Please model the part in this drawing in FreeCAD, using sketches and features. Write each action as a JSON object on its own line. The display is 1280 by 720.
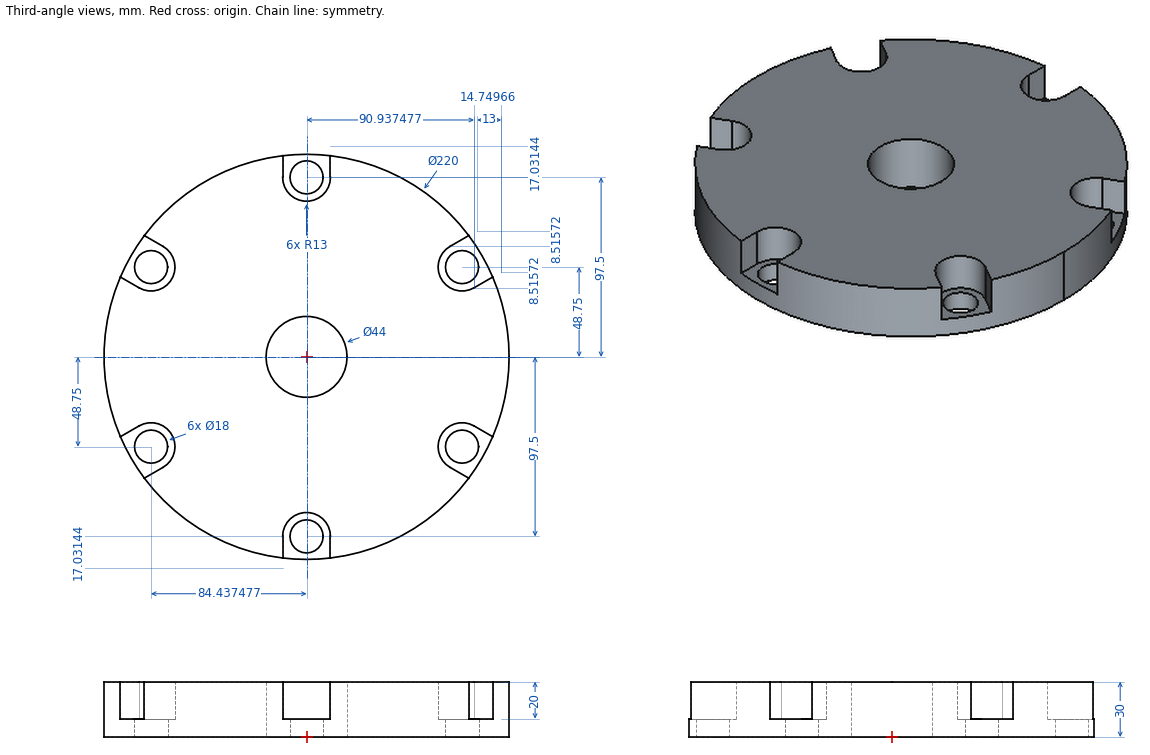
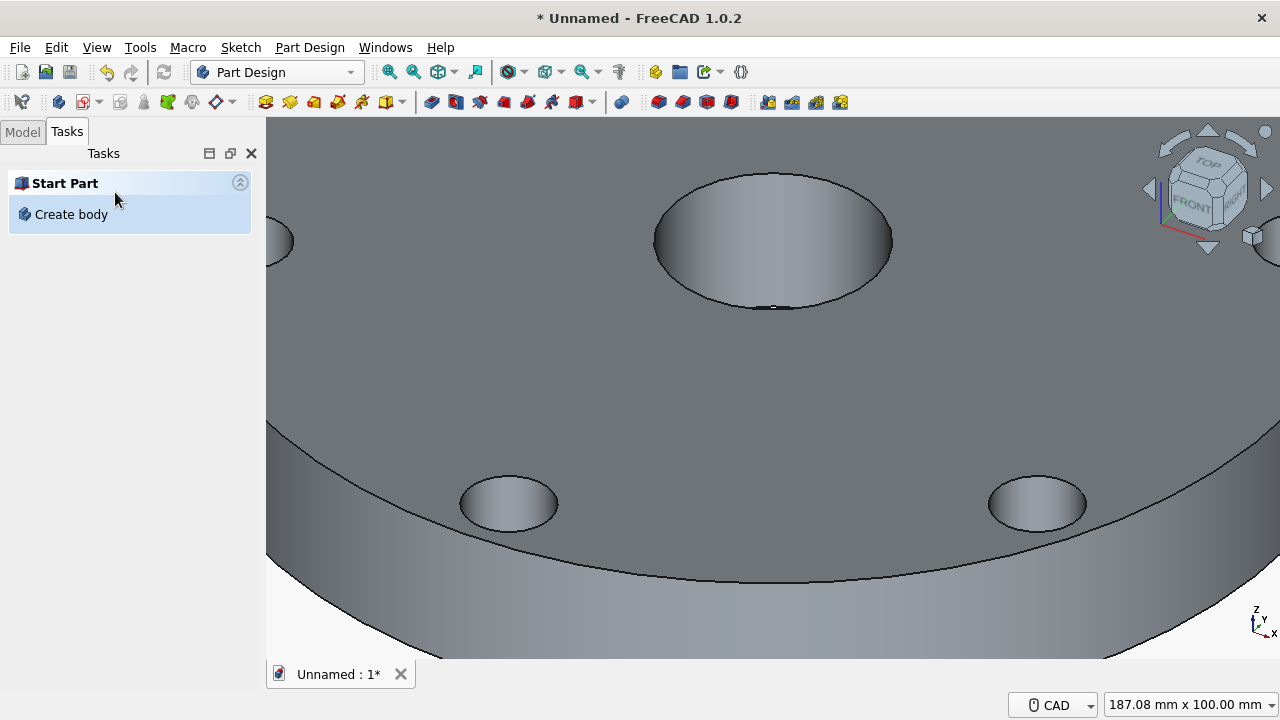
{"action": "key", "text": "v f"}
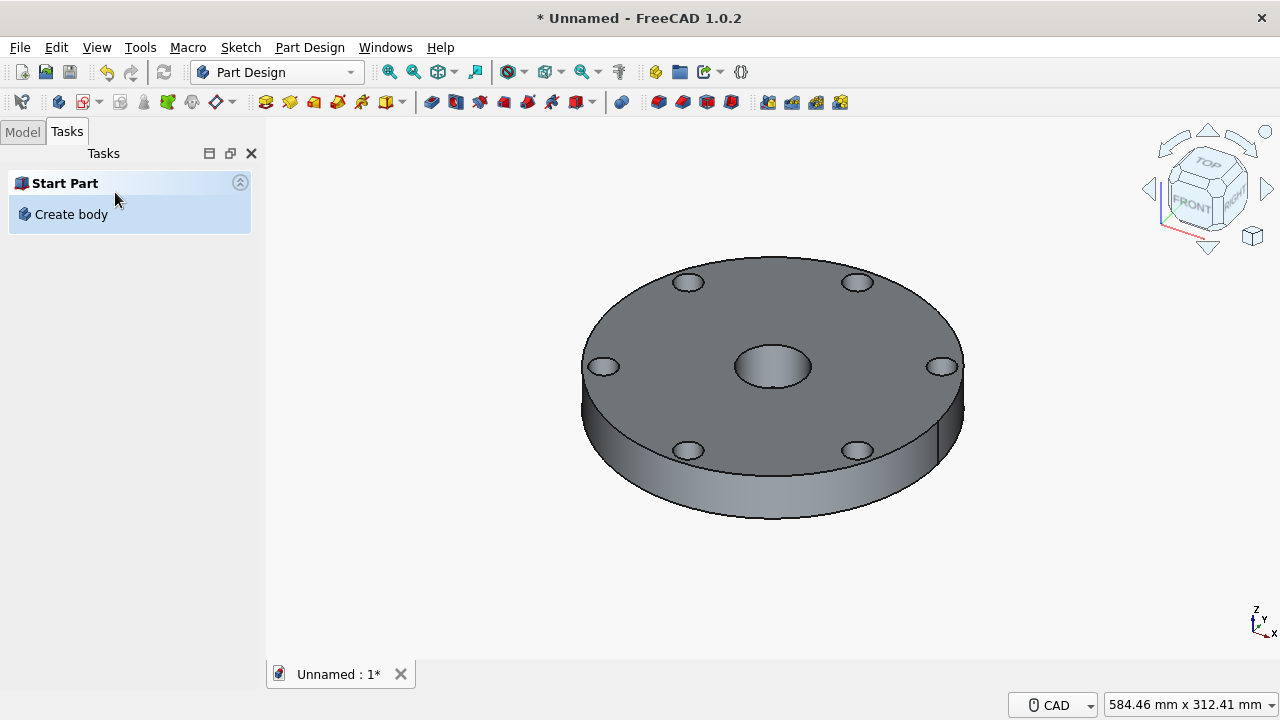
{"action": "left_click", "coordinate": [678, 334]}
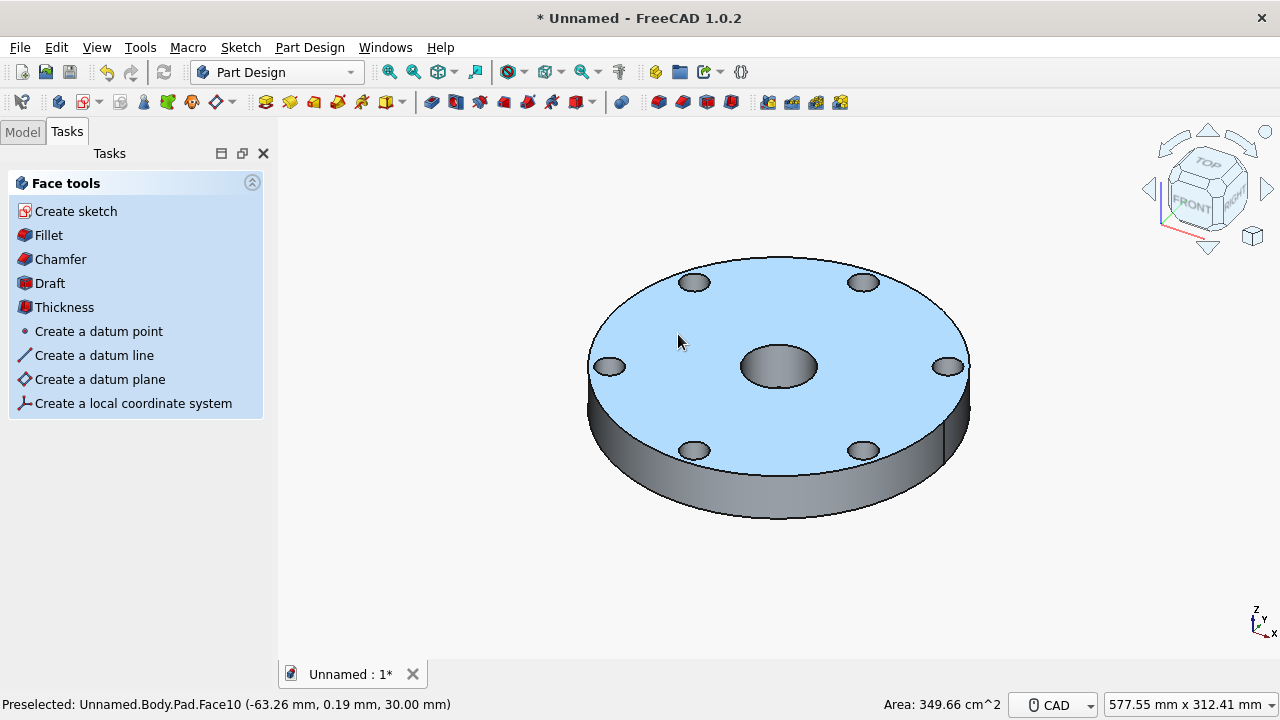
{"action": "left_click", "coordinate": [84, 102]}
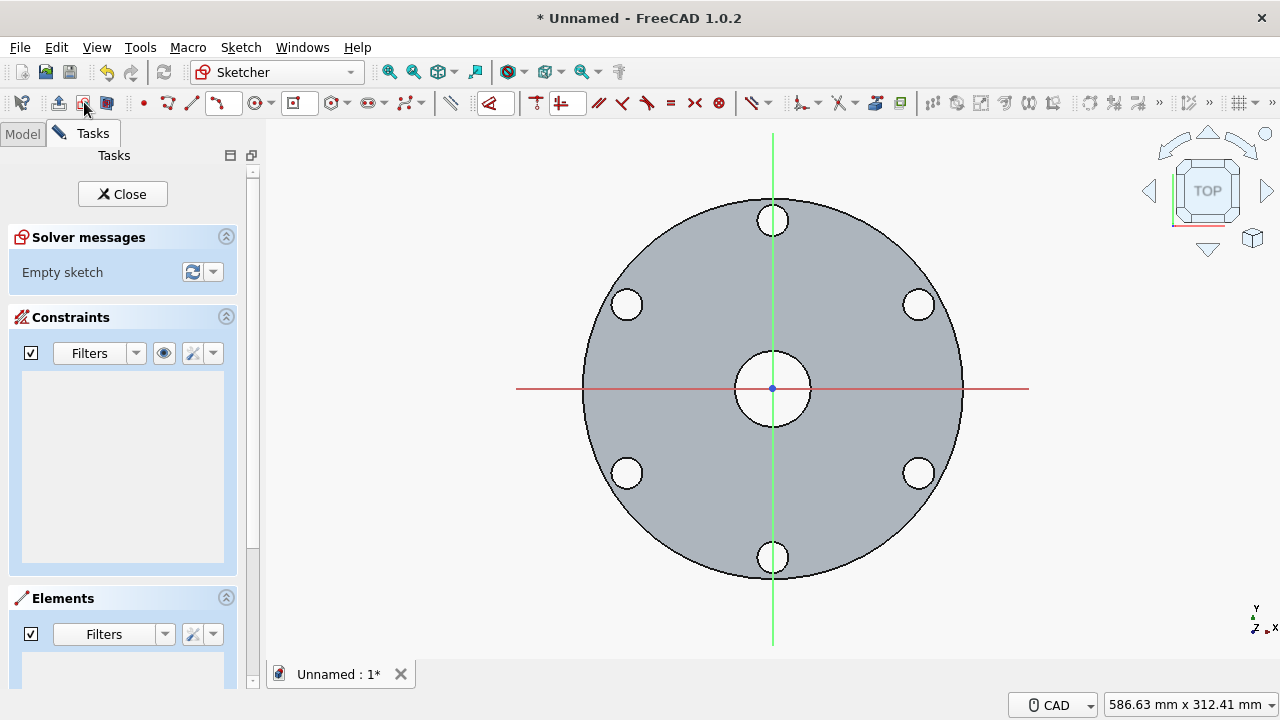
{"action": "left_click", "coordinate": [168, 104]}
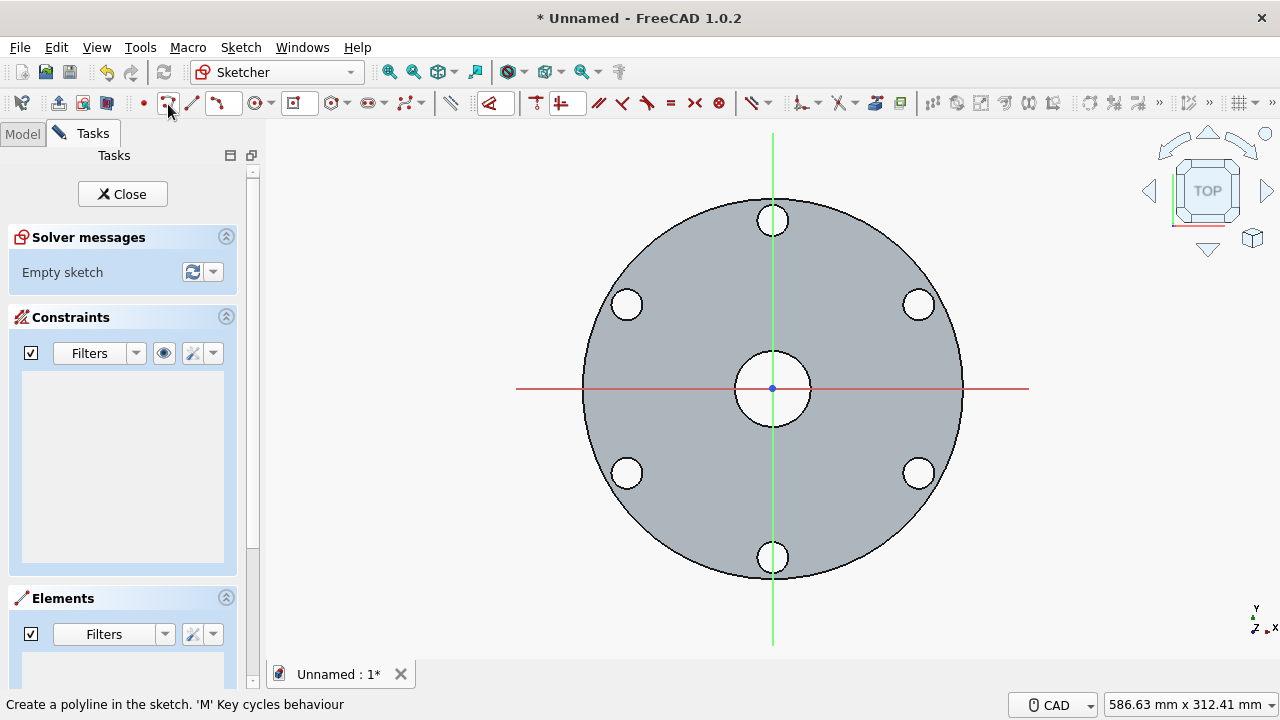
{"action": "left_click", "coordinate": [795, 220]}
{"action": "left_click", "coordinate": [795, 191]}
{"action": "left_click", "coordinate": [750, 191]}
{"action": "left_click", "coordinate": [750, 220]}
{"action": "right_click", "coordinate": [750, 220]}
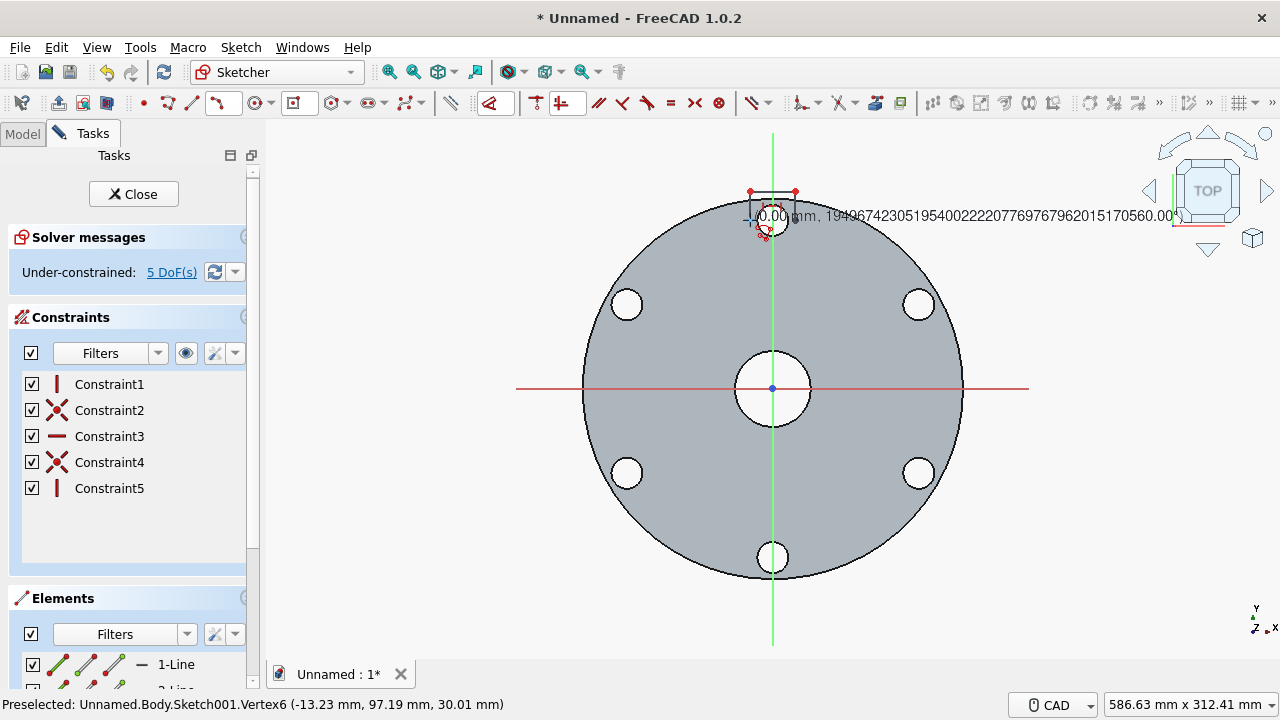
{"action": "left_click", "coordinate": [218, 104]}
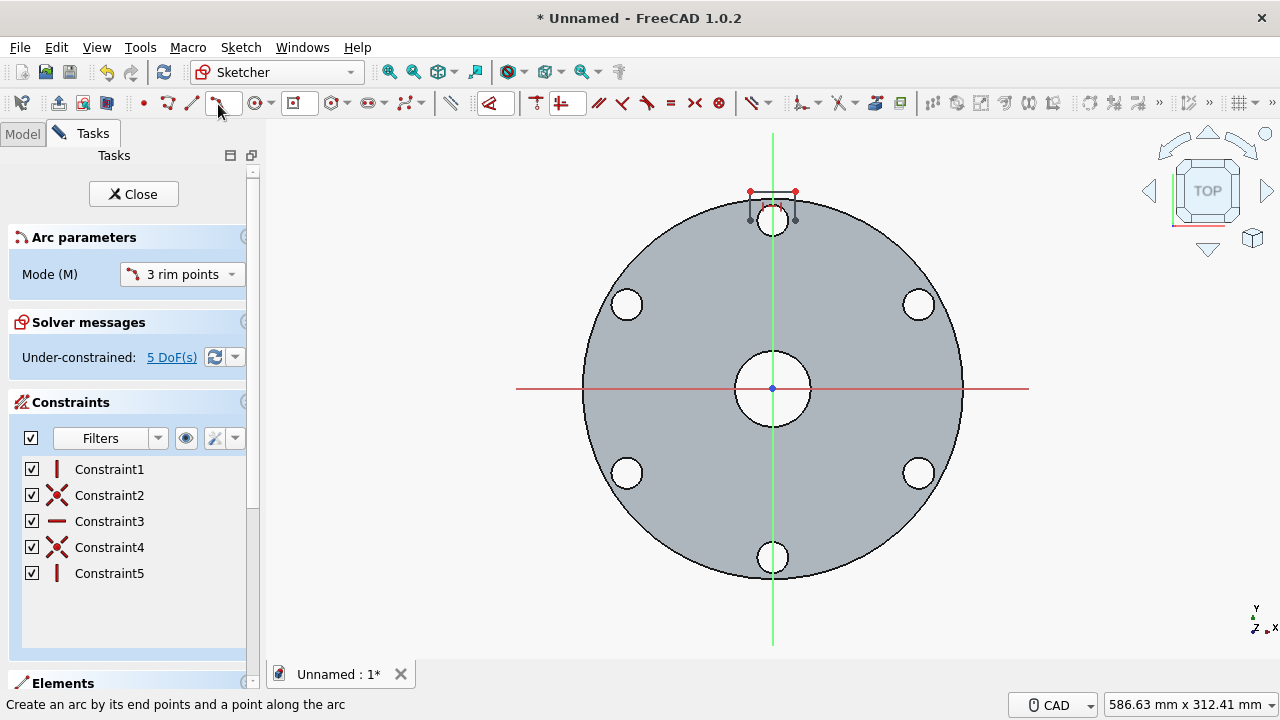
{"action": "left_click", "coordinate": [750, 221]}
{"action": "left_click", "coordinate": [795, 221]}
{"action": "left_click", "coordinate": [760, 239]}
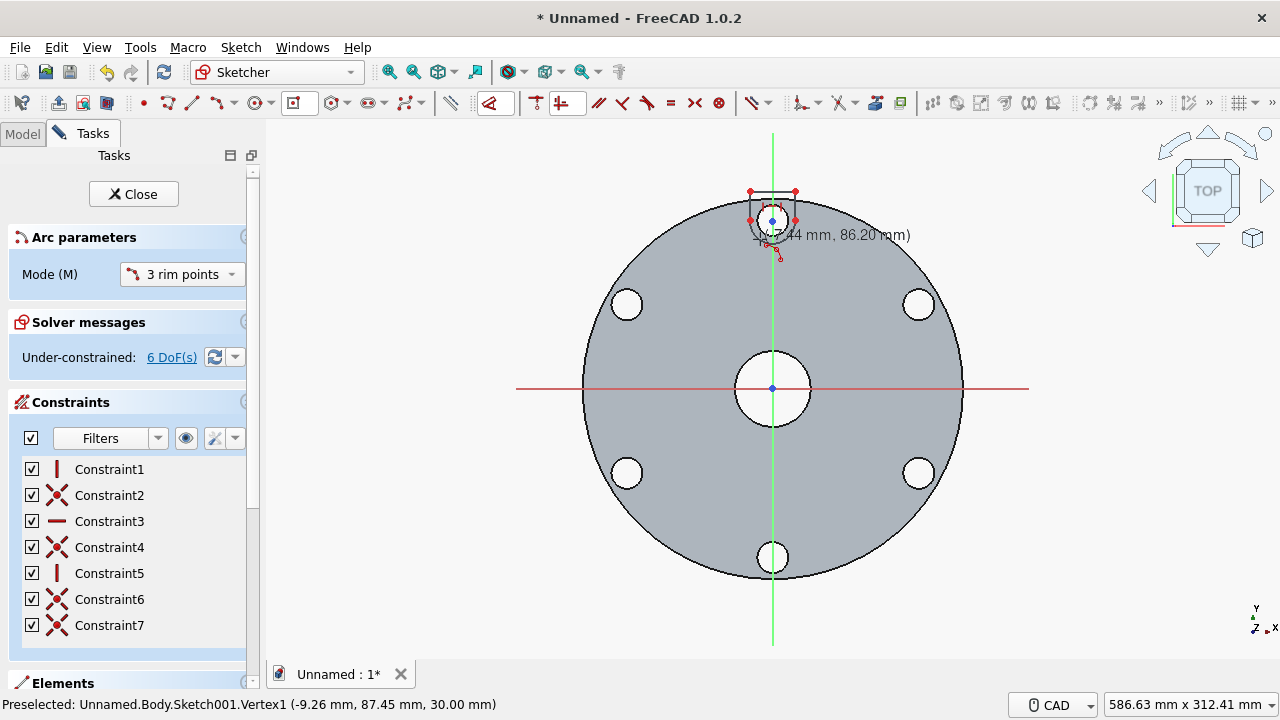
{"action": "left_click", "coordinate": [168, 104]}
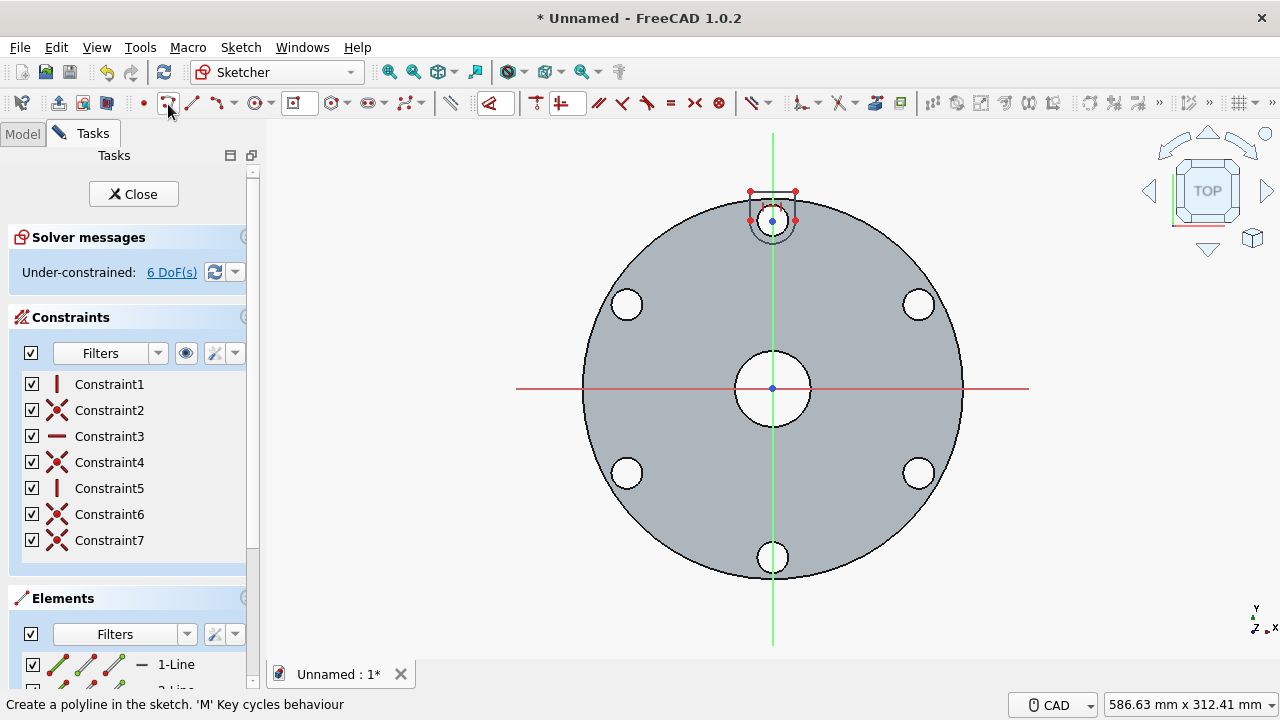
{"action": "left_click", "coordinate": [930, 324]}
{"action": "left_click", "coordinate": [956, 309]}
{"action": "left_click", "coordinate": [933, 271]}
{"action": "left_click", "coordinate": [908, 285]}
{"action": "right_click", "coordinate": [908, 285]}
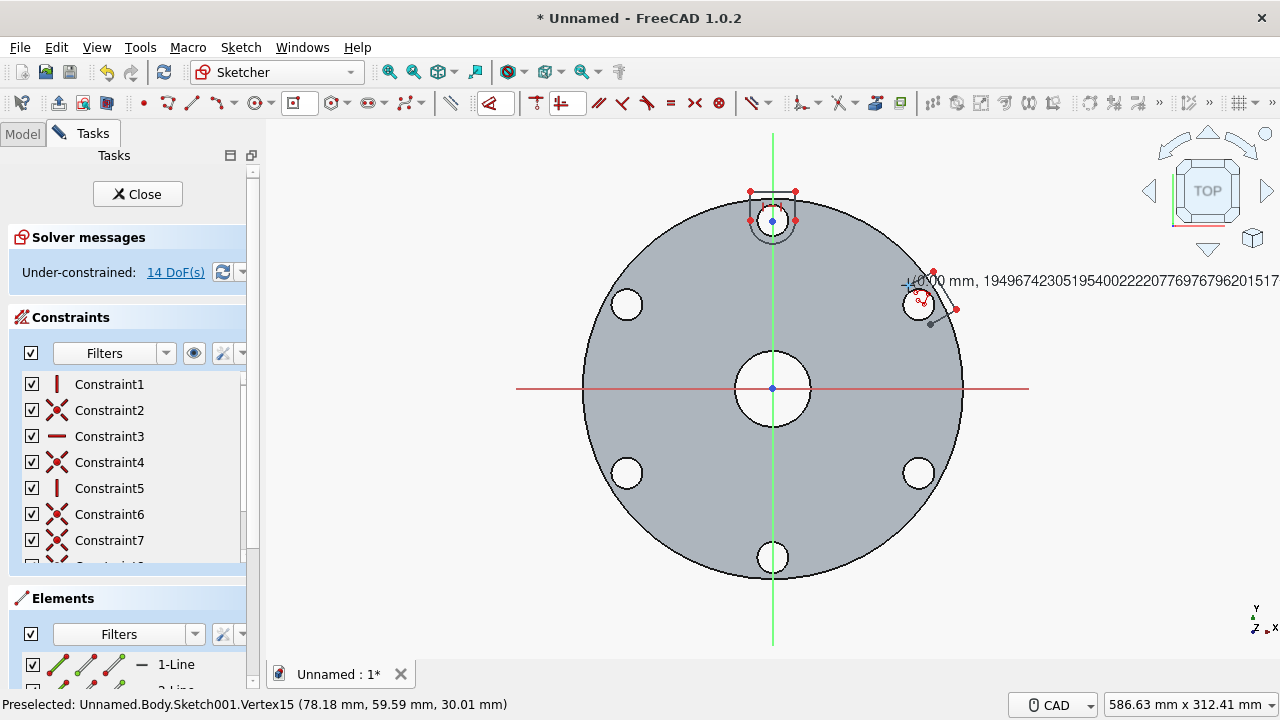
{"action": "key", "text": "g 3 a"}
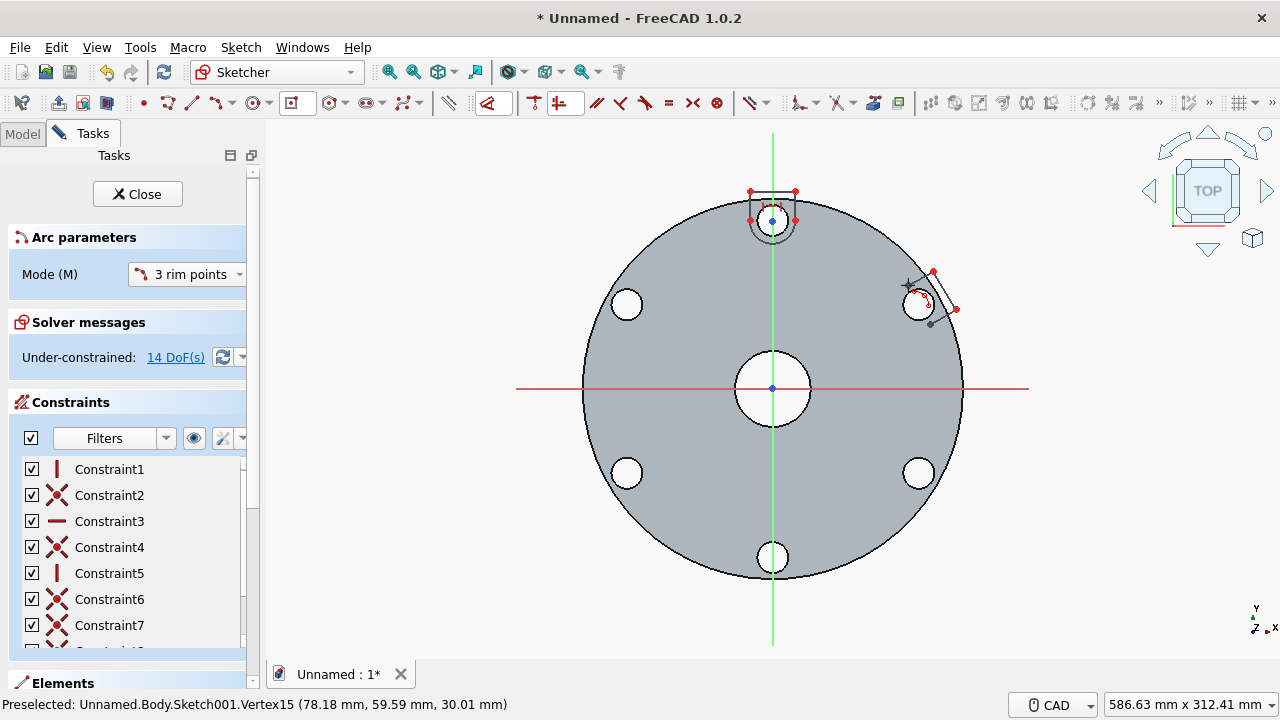
{"action": "left_click", "coordinate": [908, 286]}
{"action": "left_click", "coordinate": [930, 325]}
{"action": "left_click", "coordinate": [899, 316]}